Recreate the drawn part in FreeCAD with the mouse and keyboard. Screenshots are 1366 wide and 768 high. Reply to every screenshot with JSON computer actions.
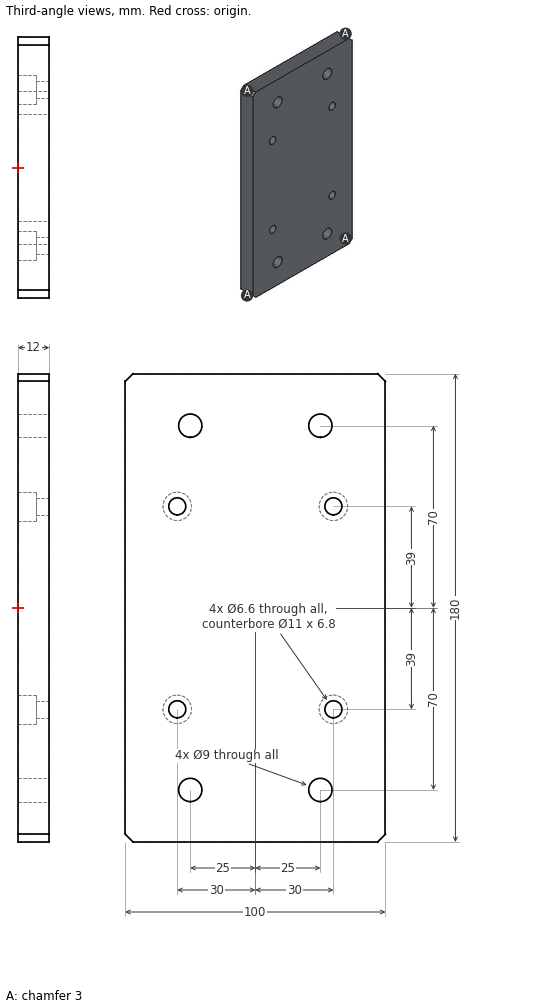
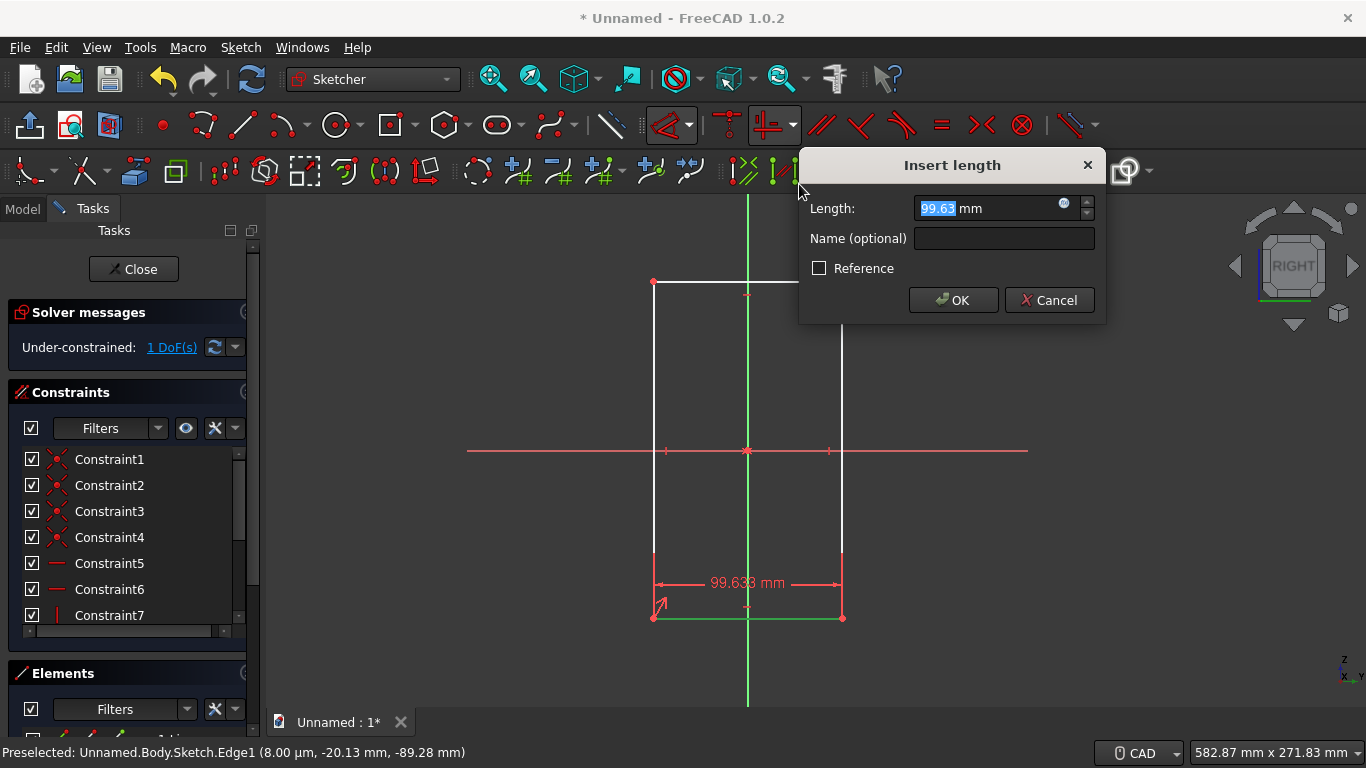
{"action": "type", "text": "100"}
{"action": "key", "text": "Return"}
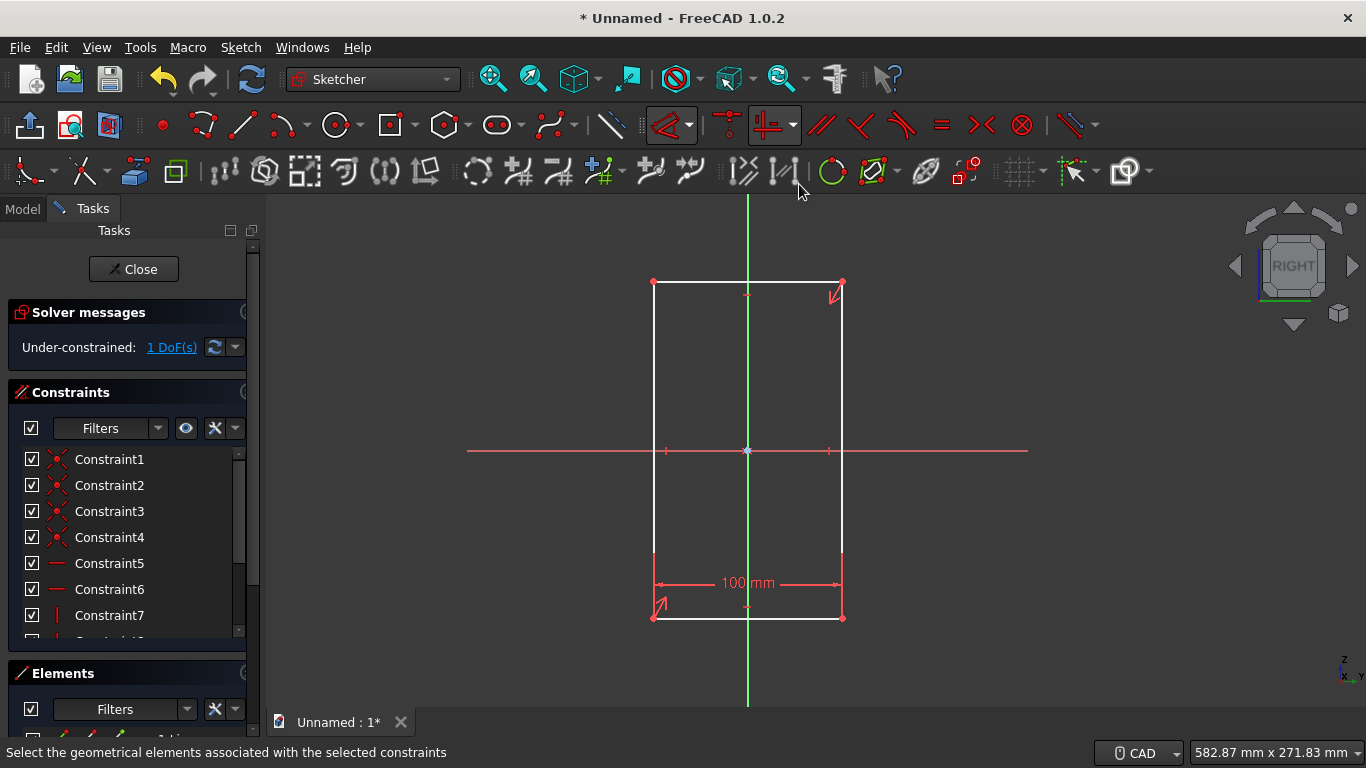
{"action": "left_click", "coordinate": [842, 518]}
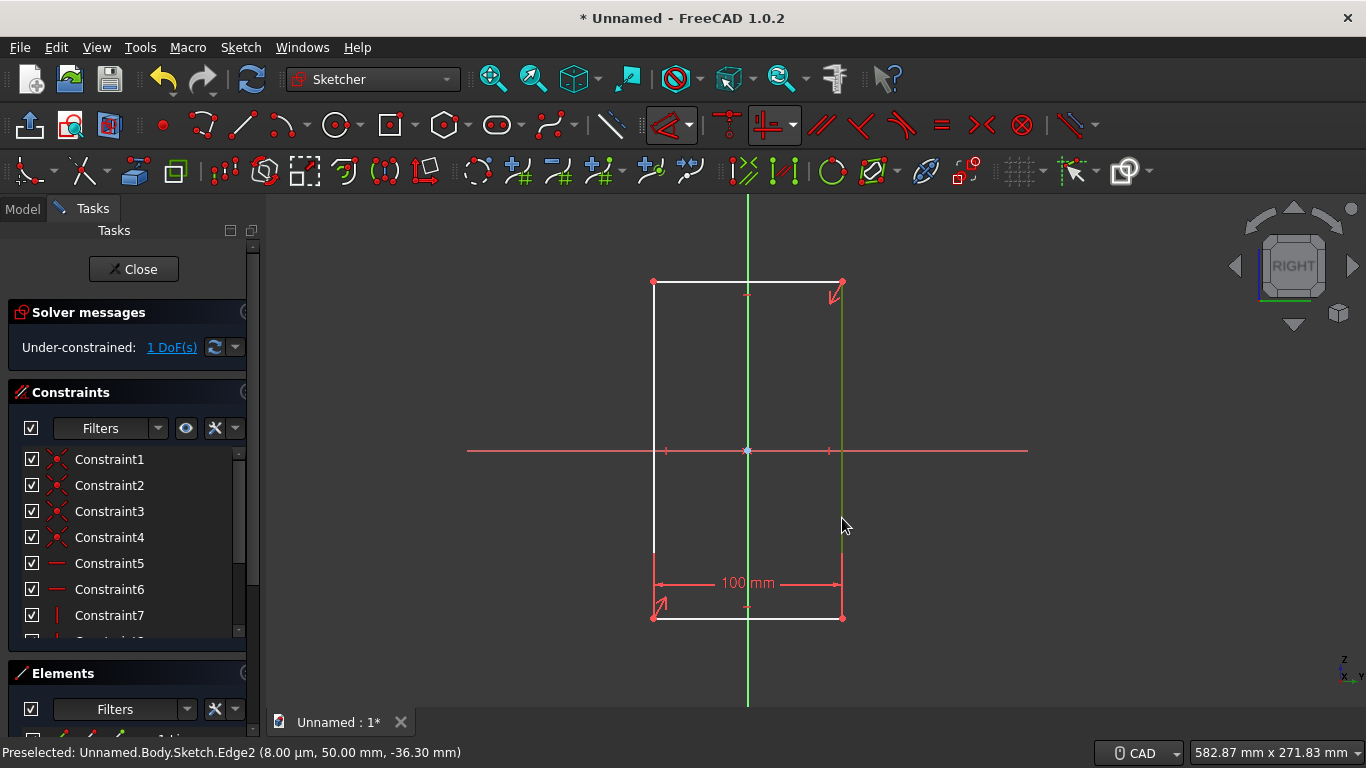
{"action": "key", "text": "i"}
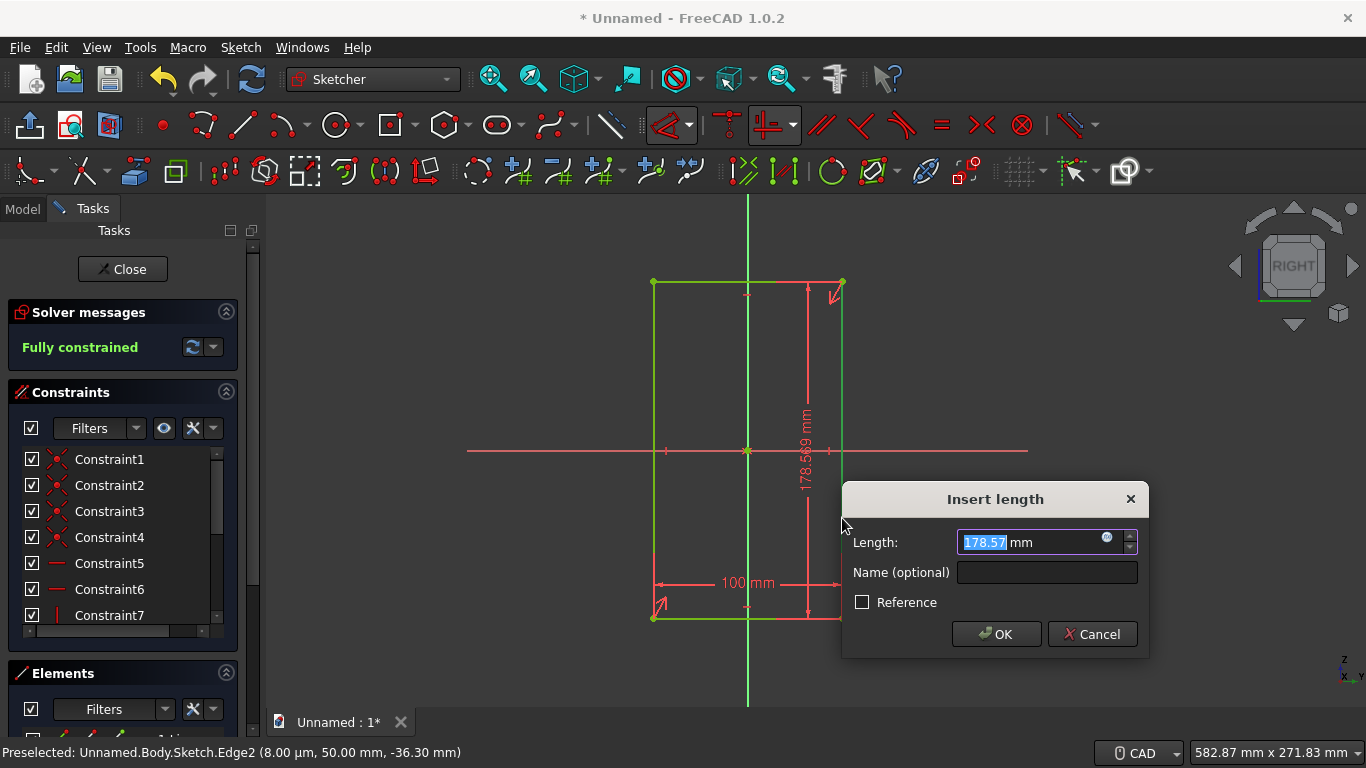
{"action": "type", "text": "180"}
{"action": "key", "text": "Return"}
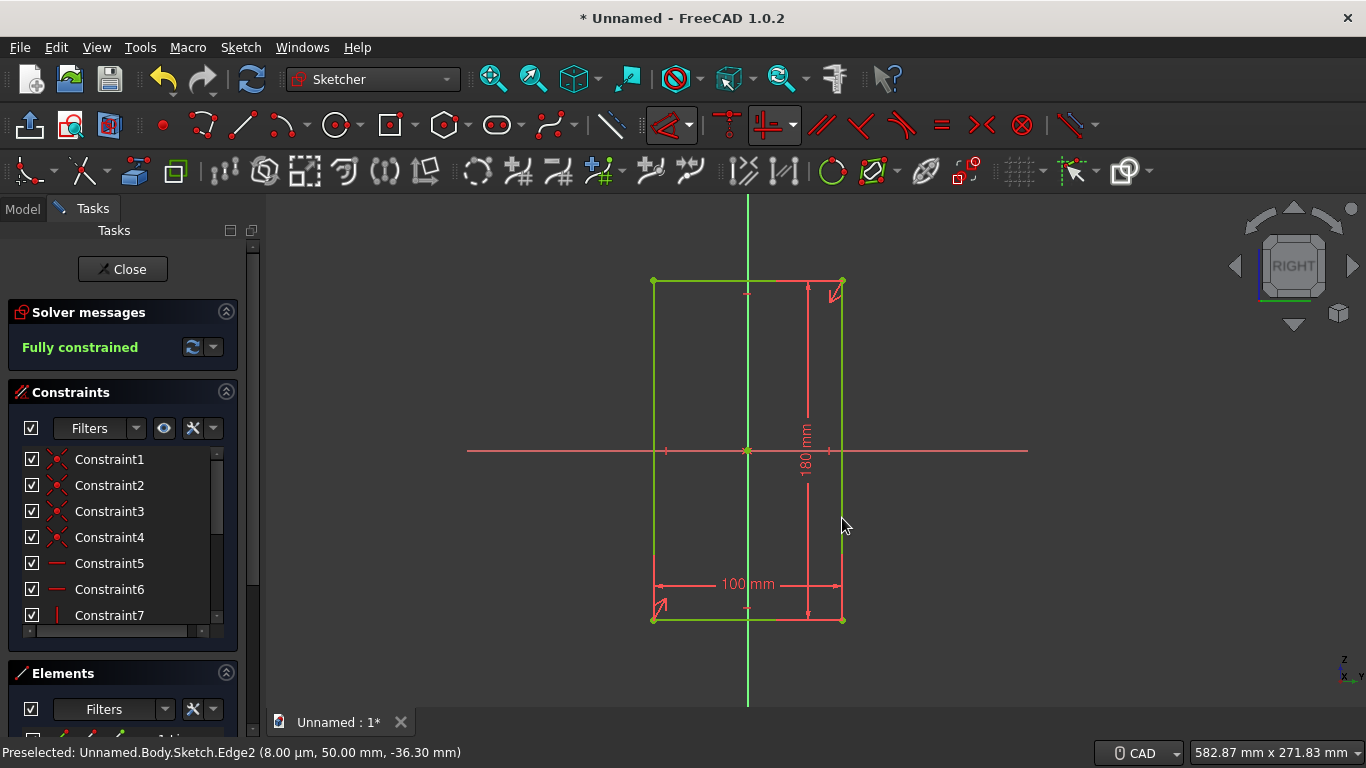
{"action": "left_click", "coordinate": [123, 269]}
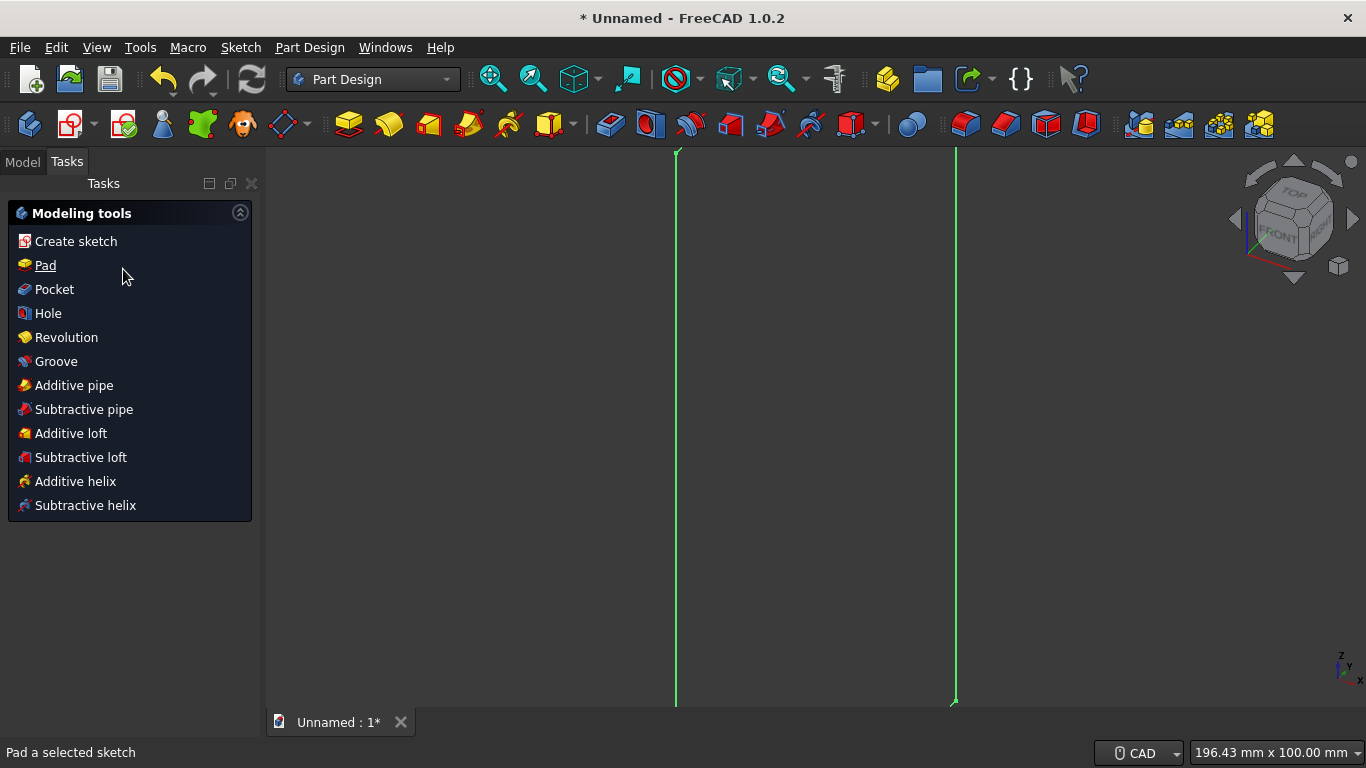
{"action": "left_click", "coordinate": [350, 124]}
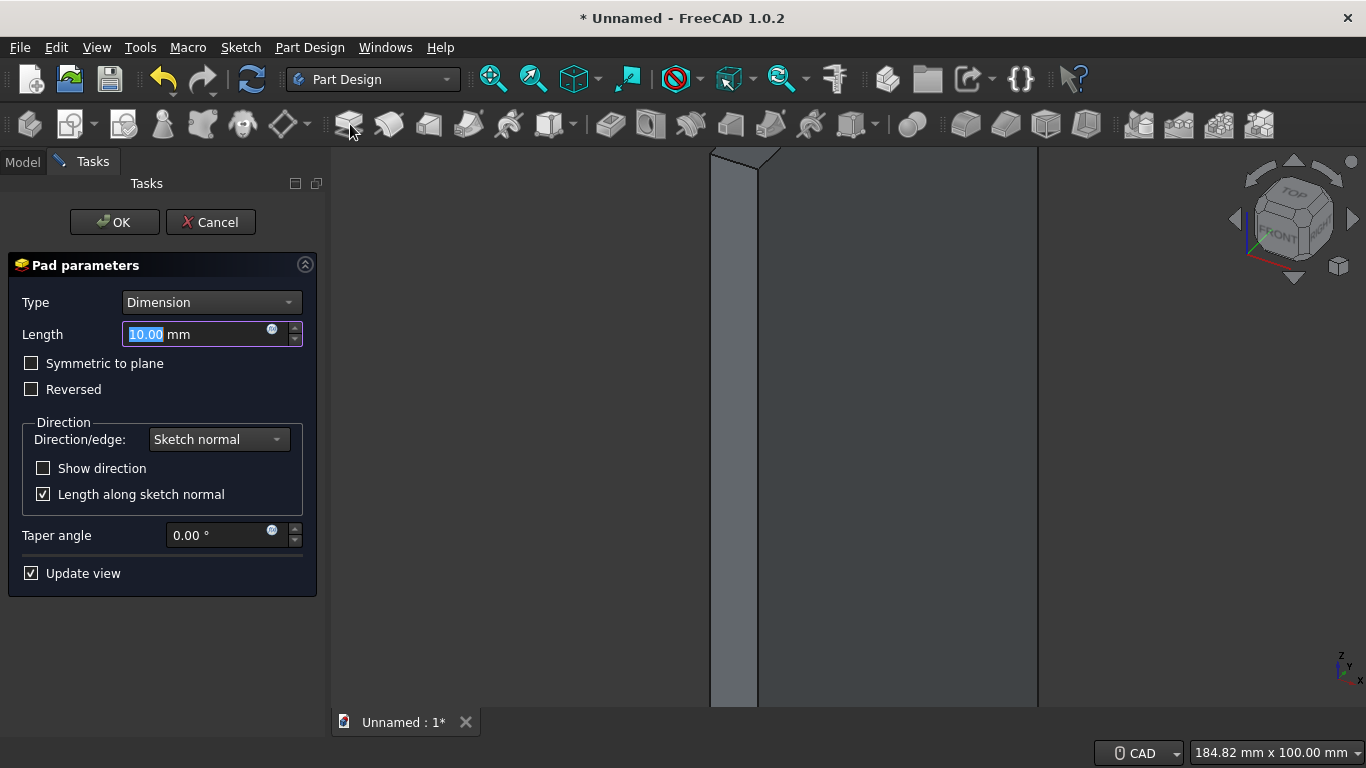
{"action": "type", "text": "12"}
{"action": "key", "text": "Tab"}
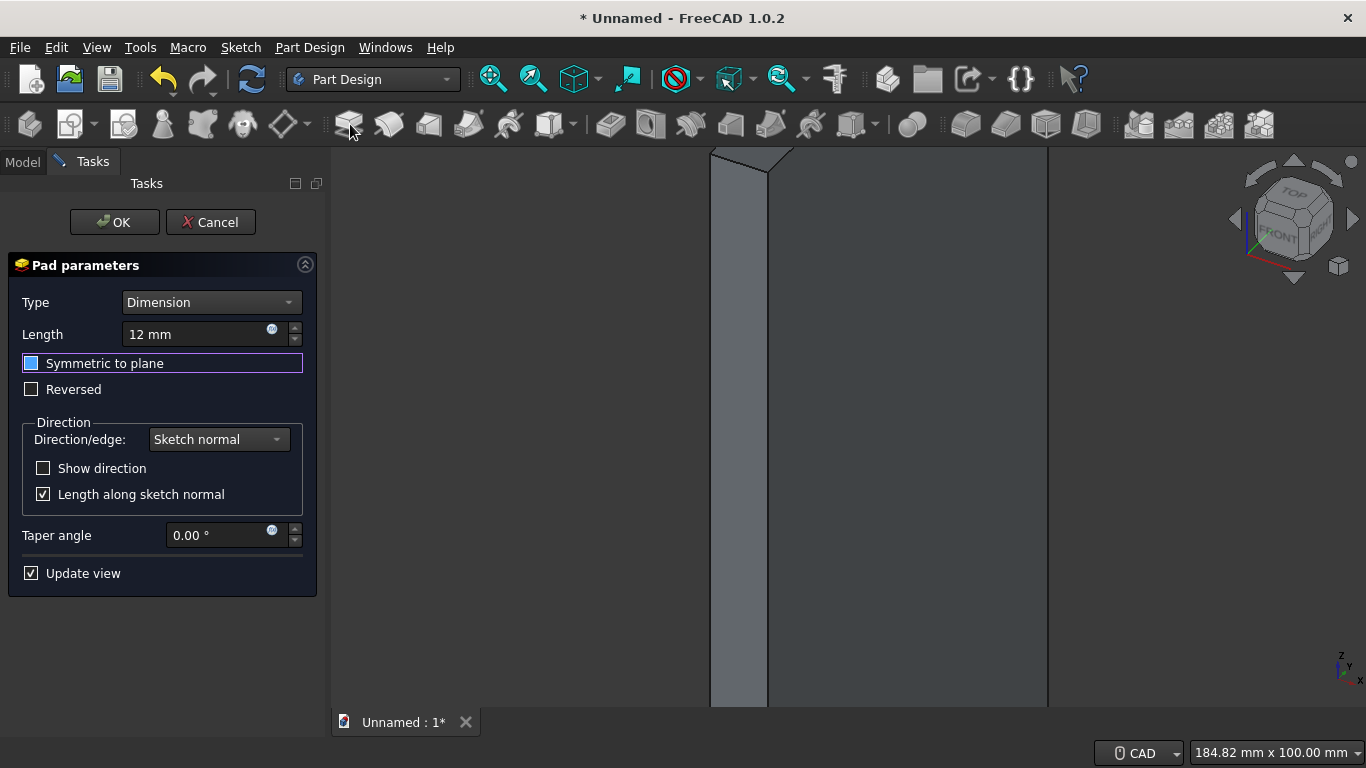
{"action": "left_click", "coordinate": [115, 222]}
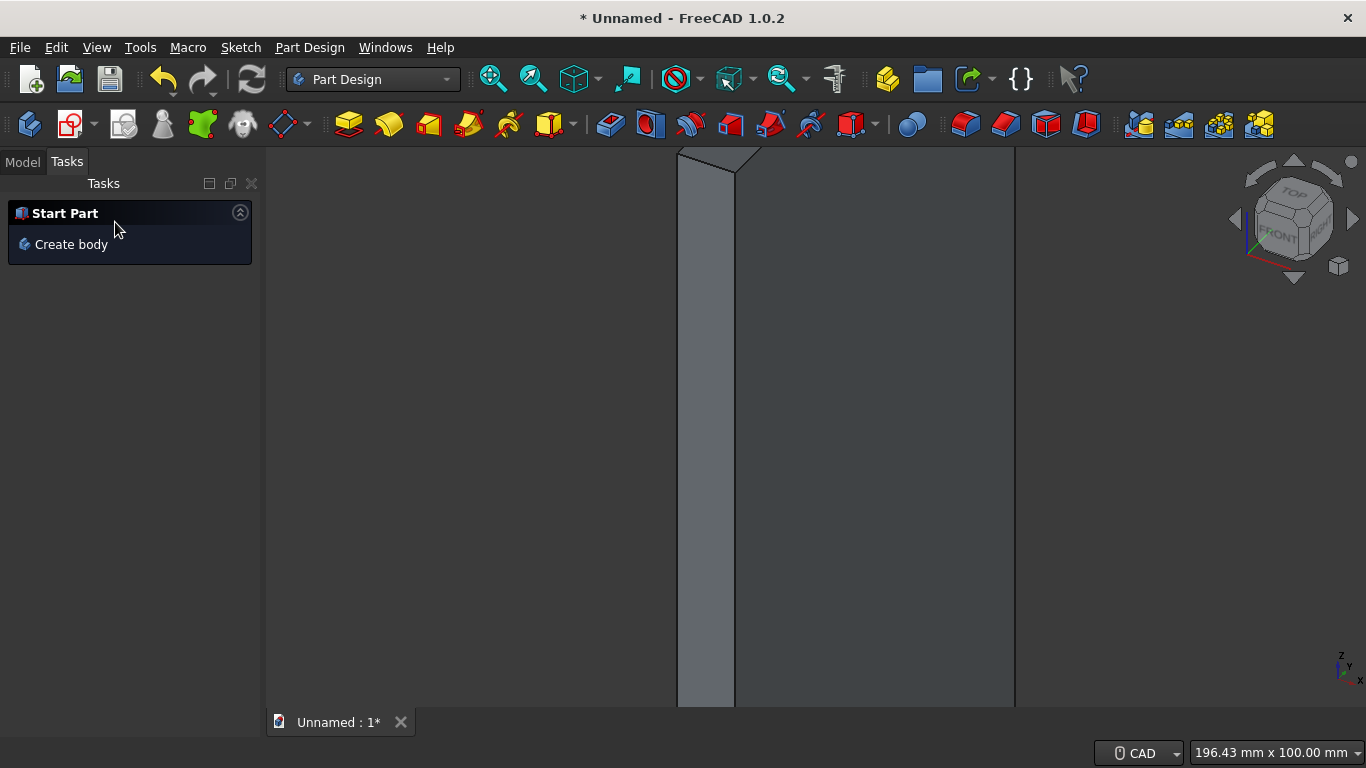
{"action": "left_click", "coordinate": [494, 80]}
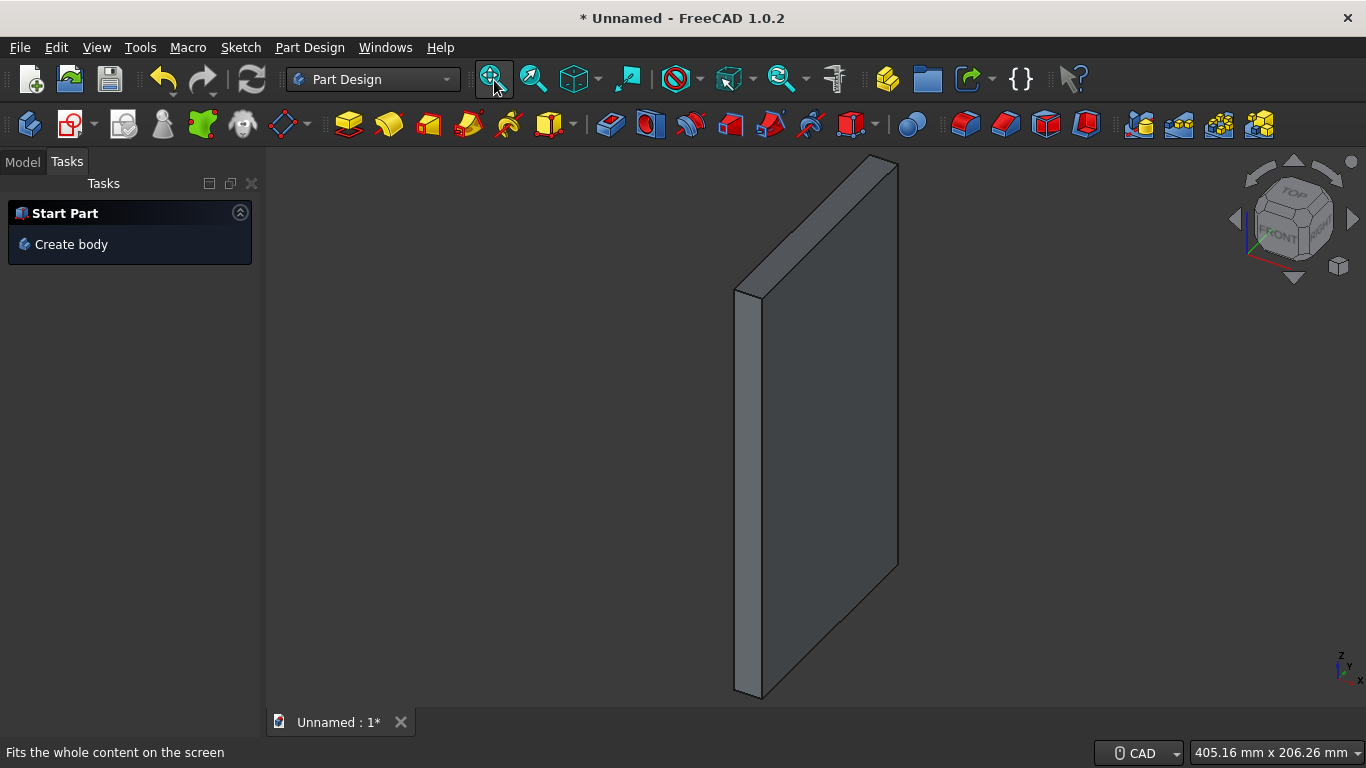
{"action": "key", "text": "6"}